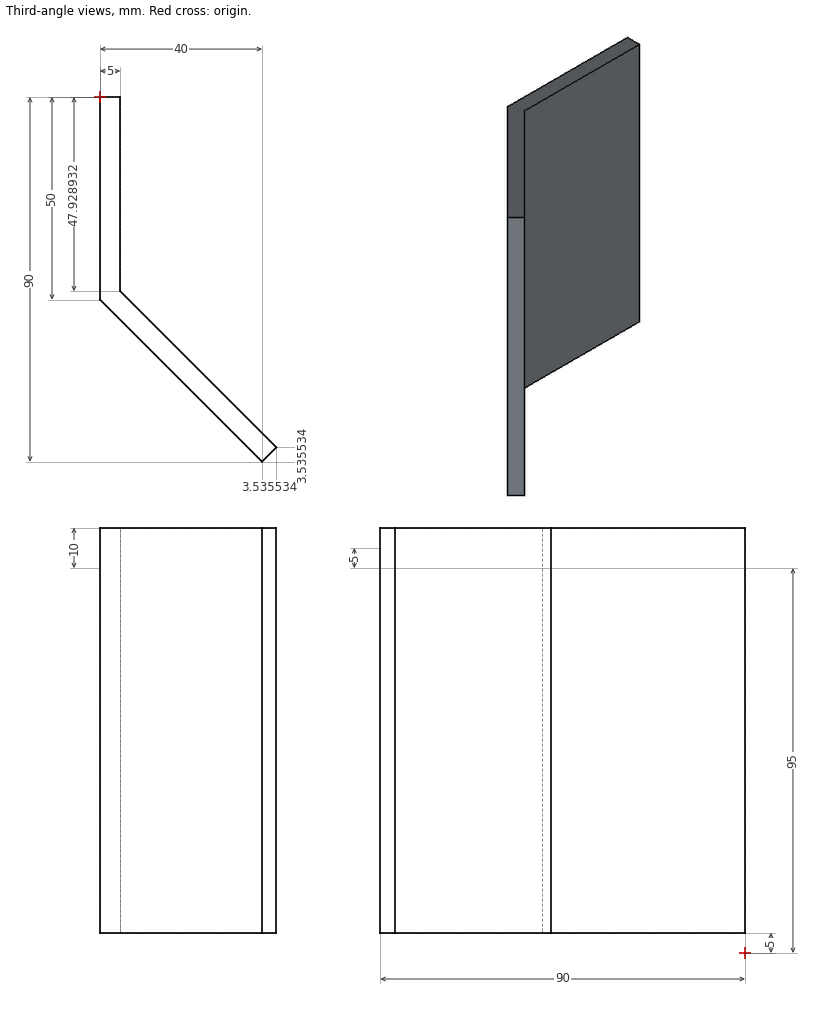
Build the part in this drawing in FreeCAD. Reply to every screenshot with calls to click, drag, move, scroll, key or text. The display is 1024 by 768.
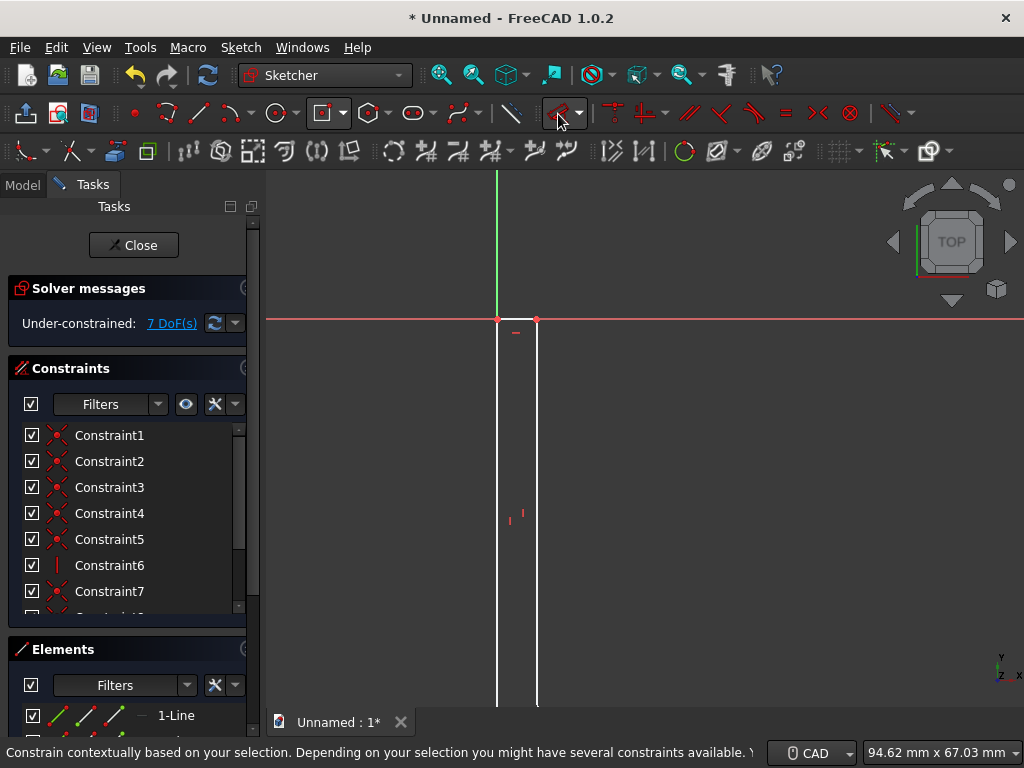
click(525, 319)
click(517, 285)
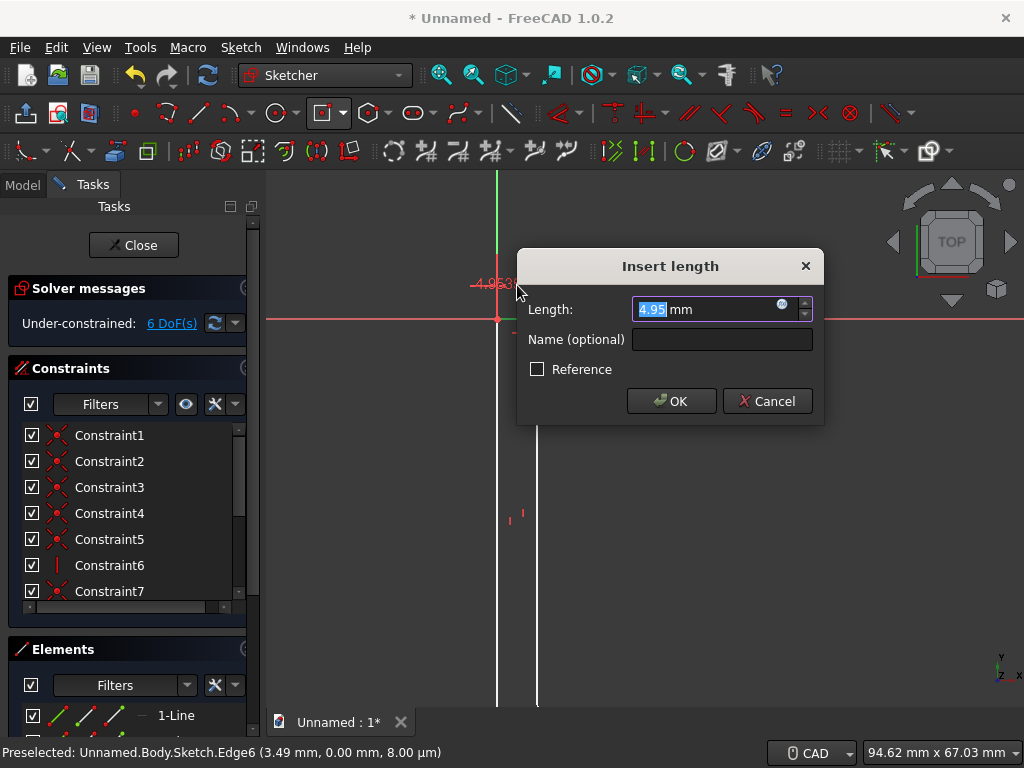
text(5)
key(Return)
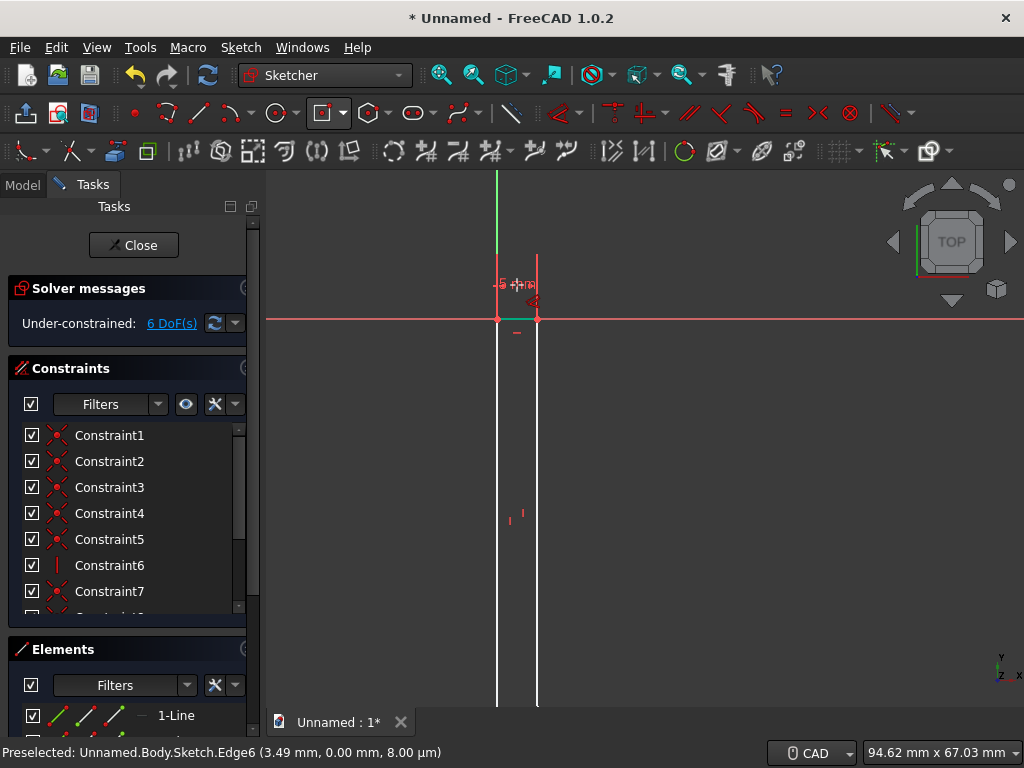
click(497, 440)
click(463, 499)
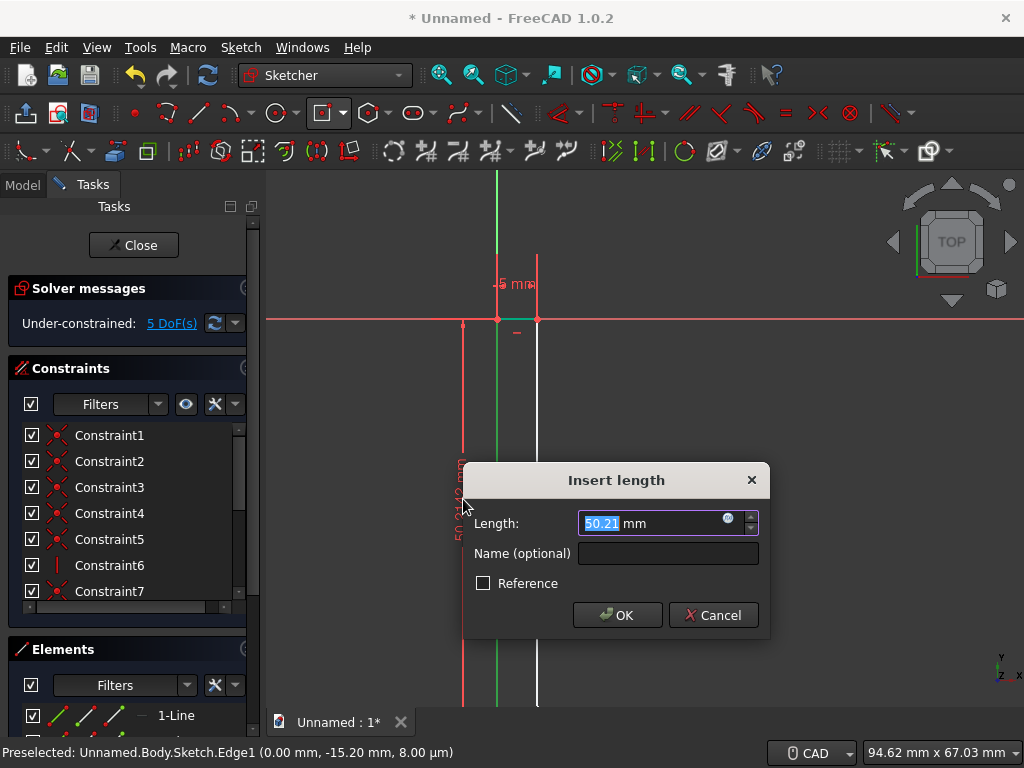
text(50)
key(Return)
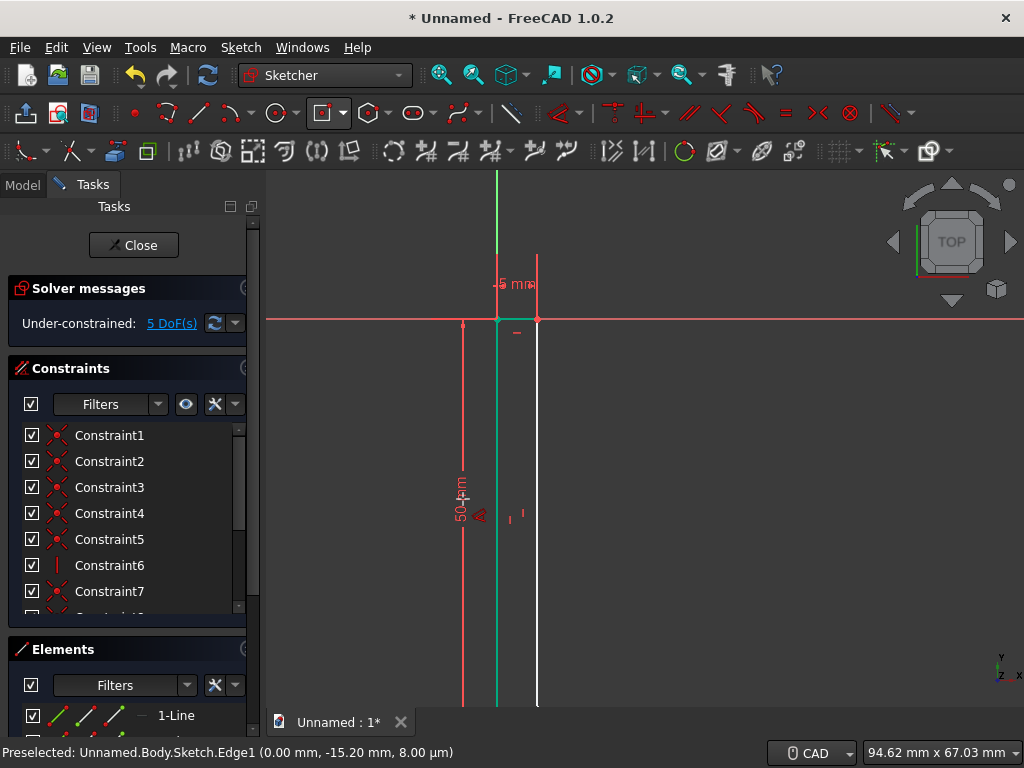
scroll(499, 242, down, 4)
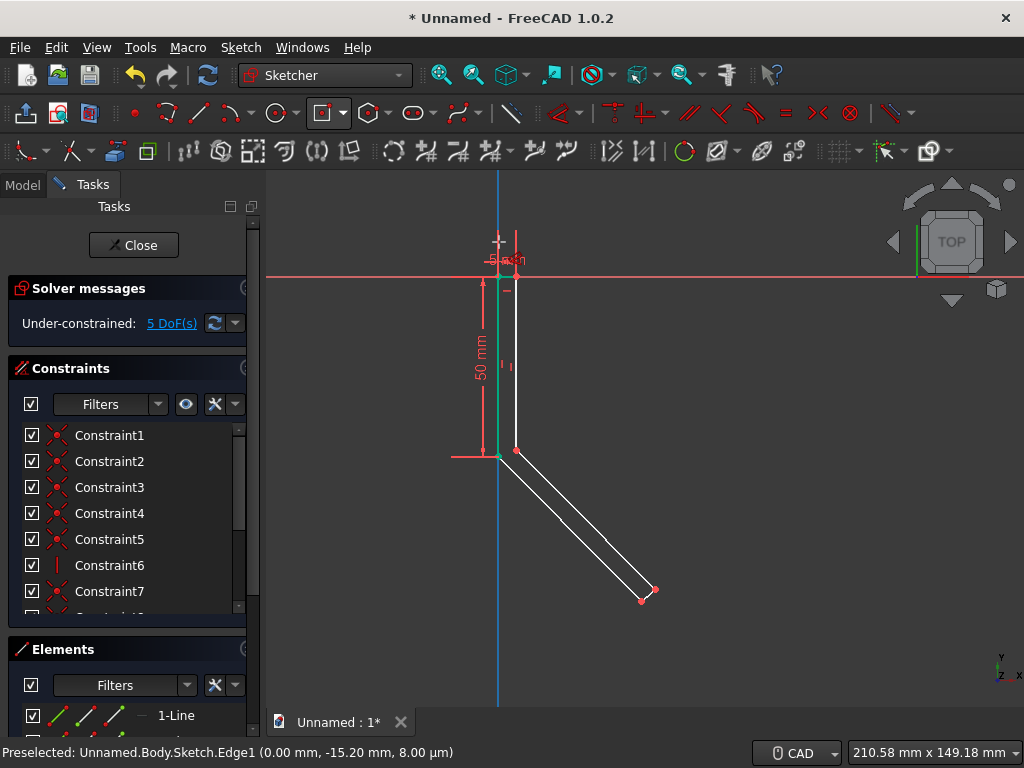
click(642, 602)
click(570, 636)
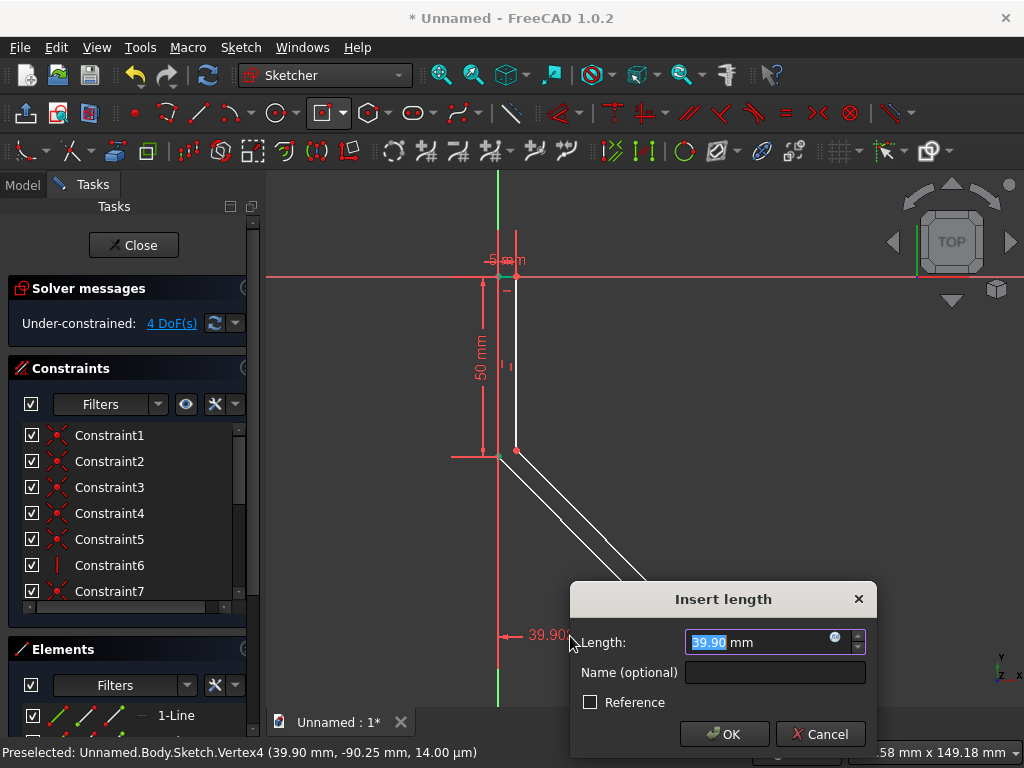
text(40)
key(Return)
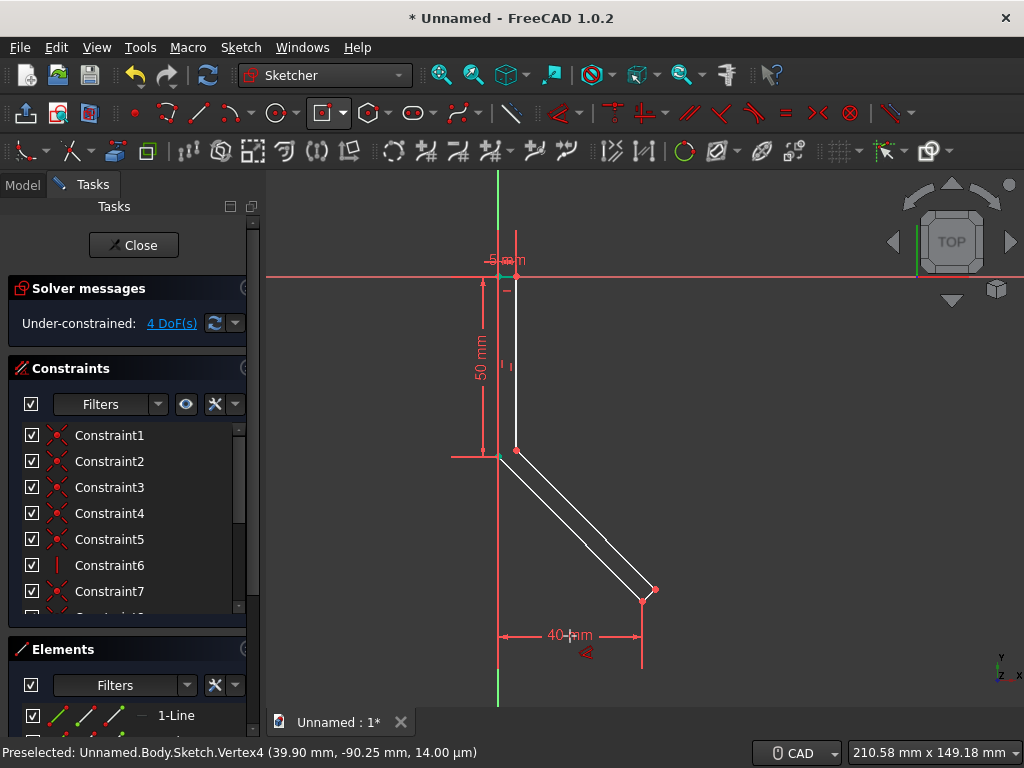
click(642, 602)
click(464, 439)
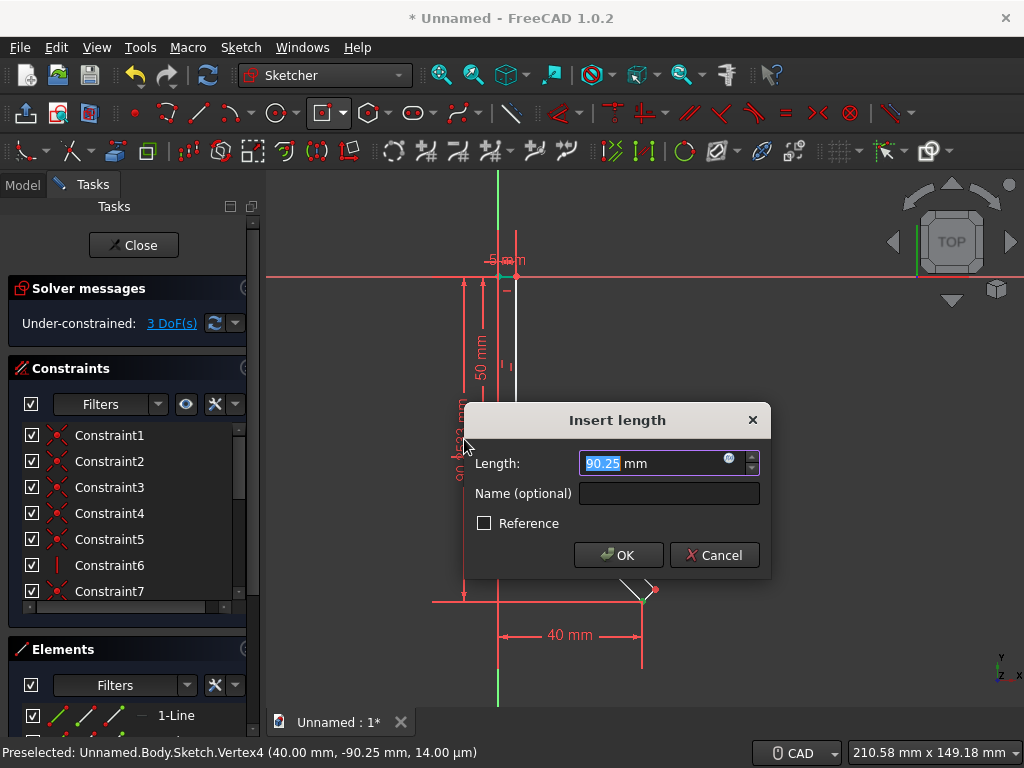
text(90)
key(Return)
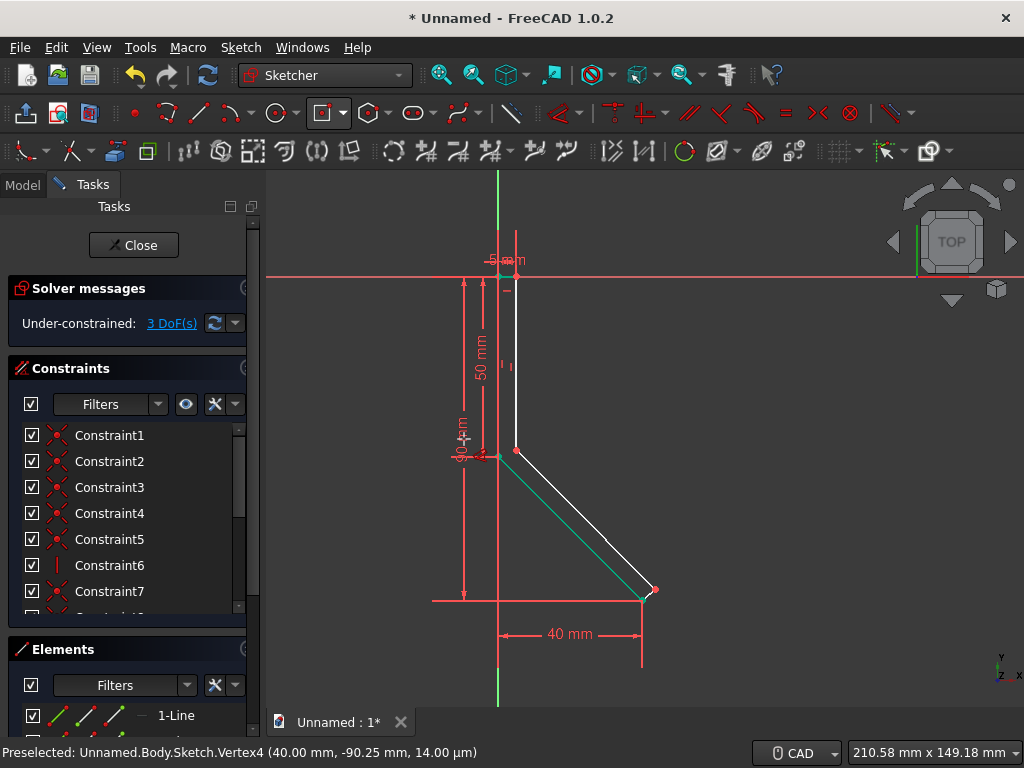
click(516, 398)
click(482, 324)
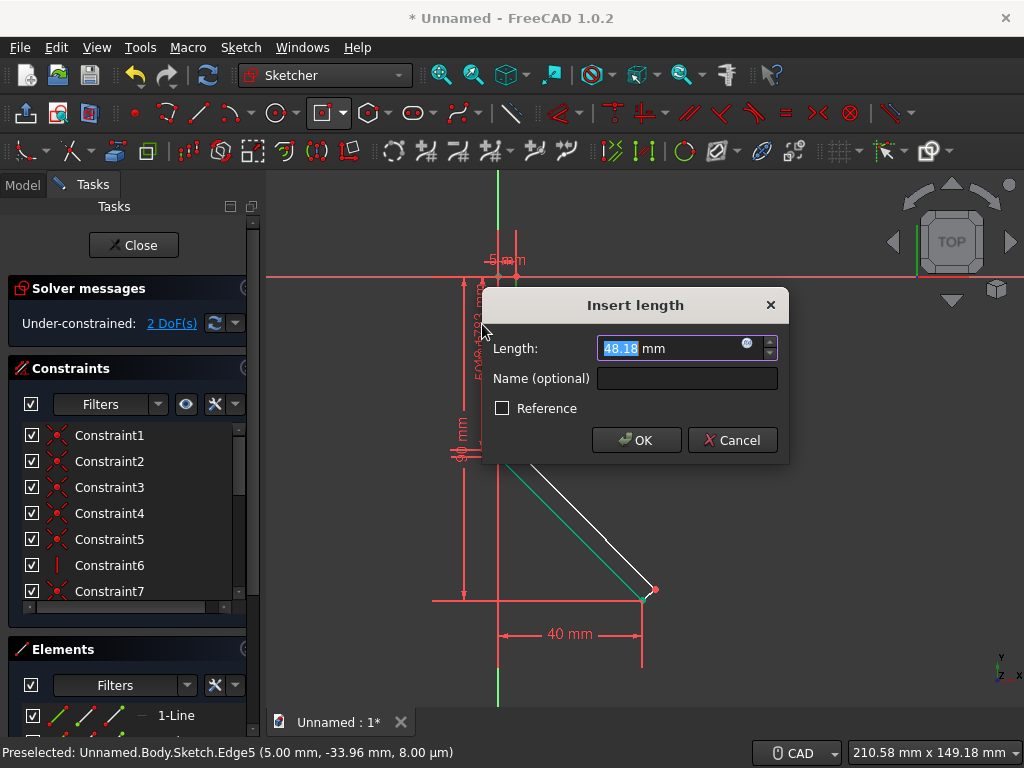
text(47.928932)
key(Return)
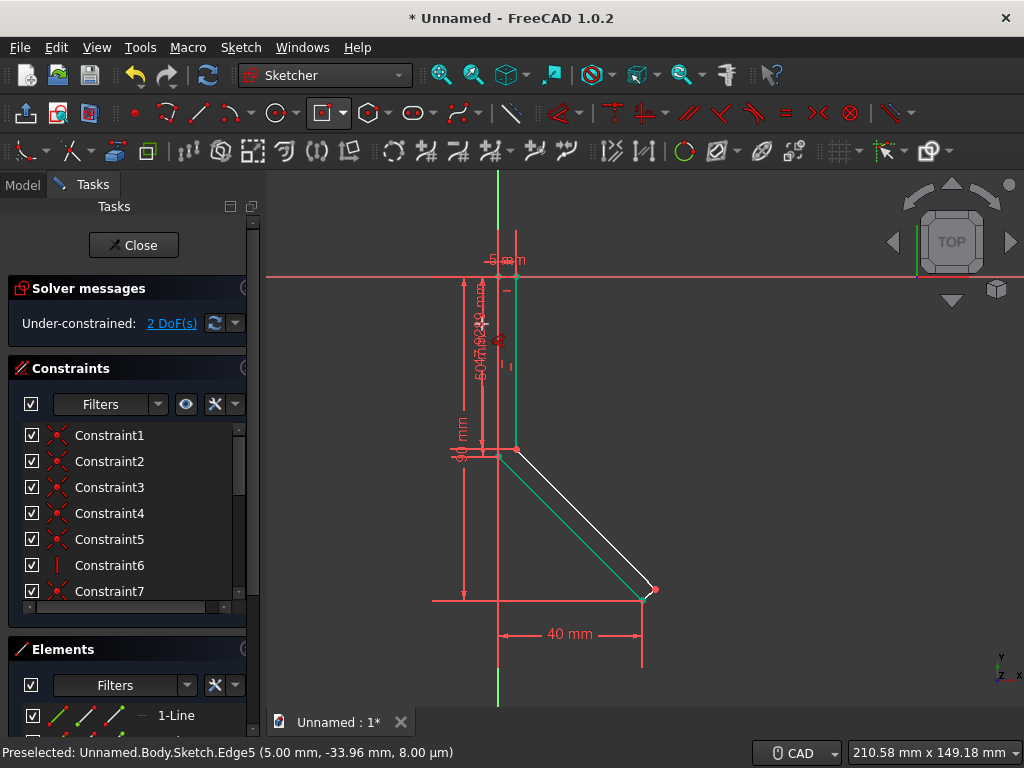
scroll(649, 595, up, 6)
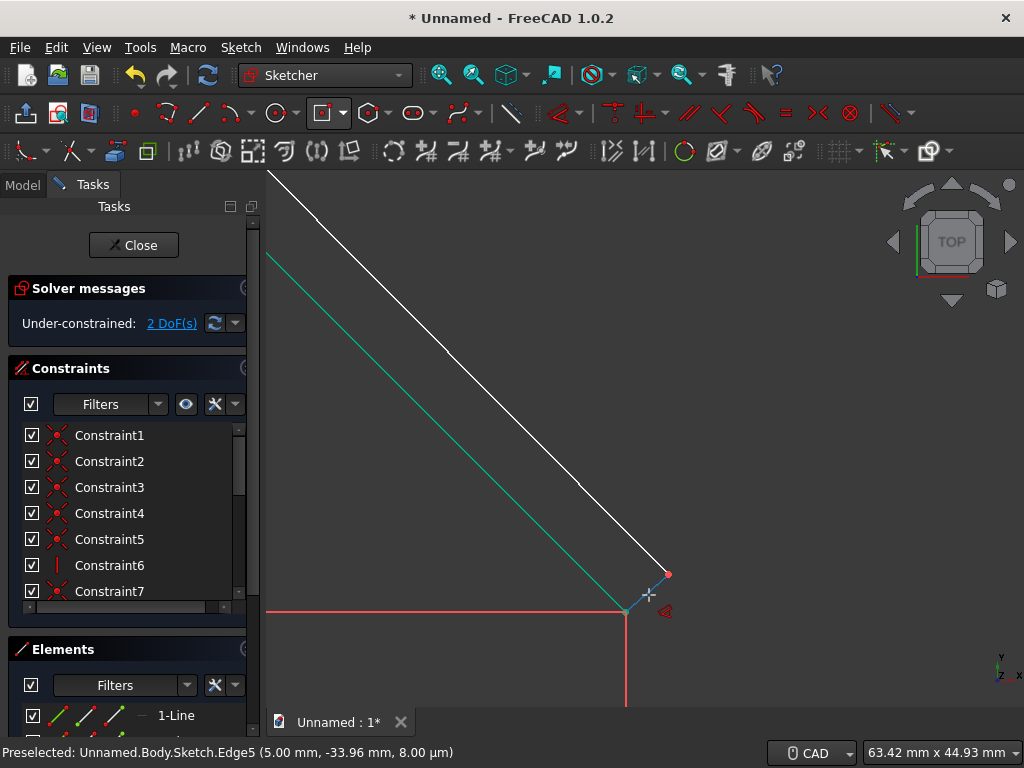
click(647, 593)
click(647, 646)